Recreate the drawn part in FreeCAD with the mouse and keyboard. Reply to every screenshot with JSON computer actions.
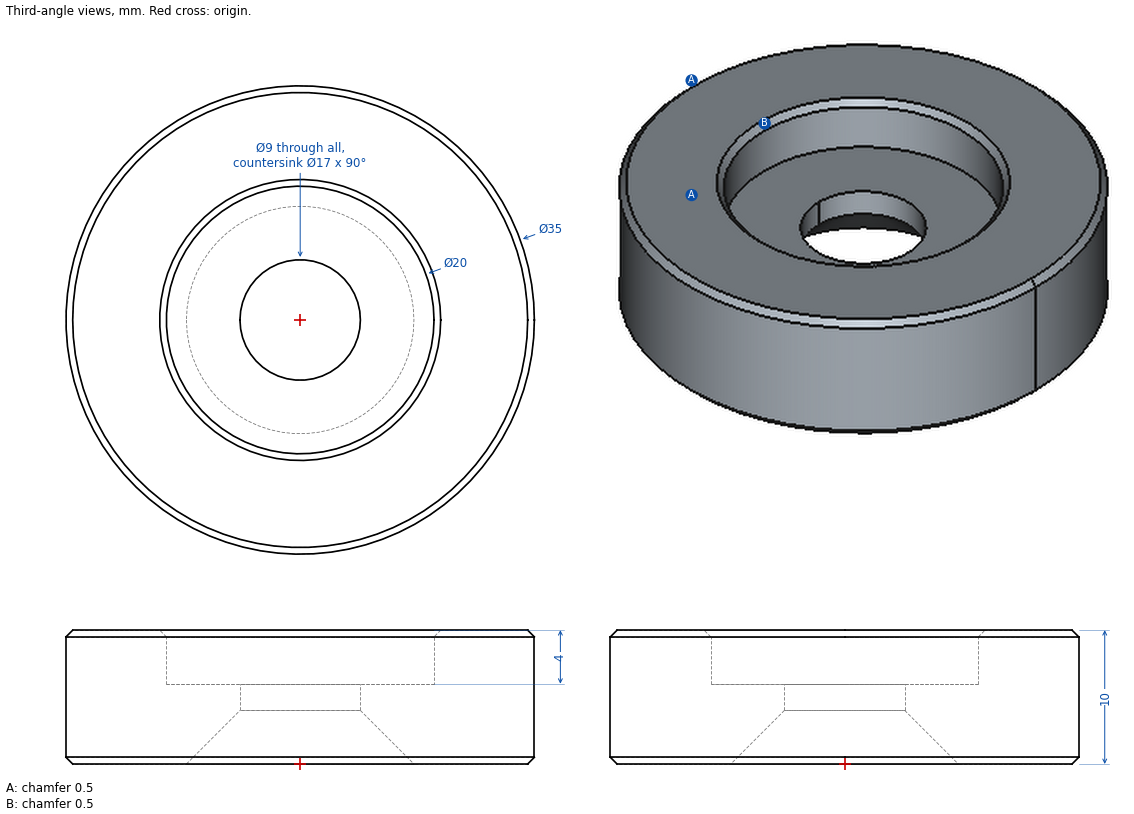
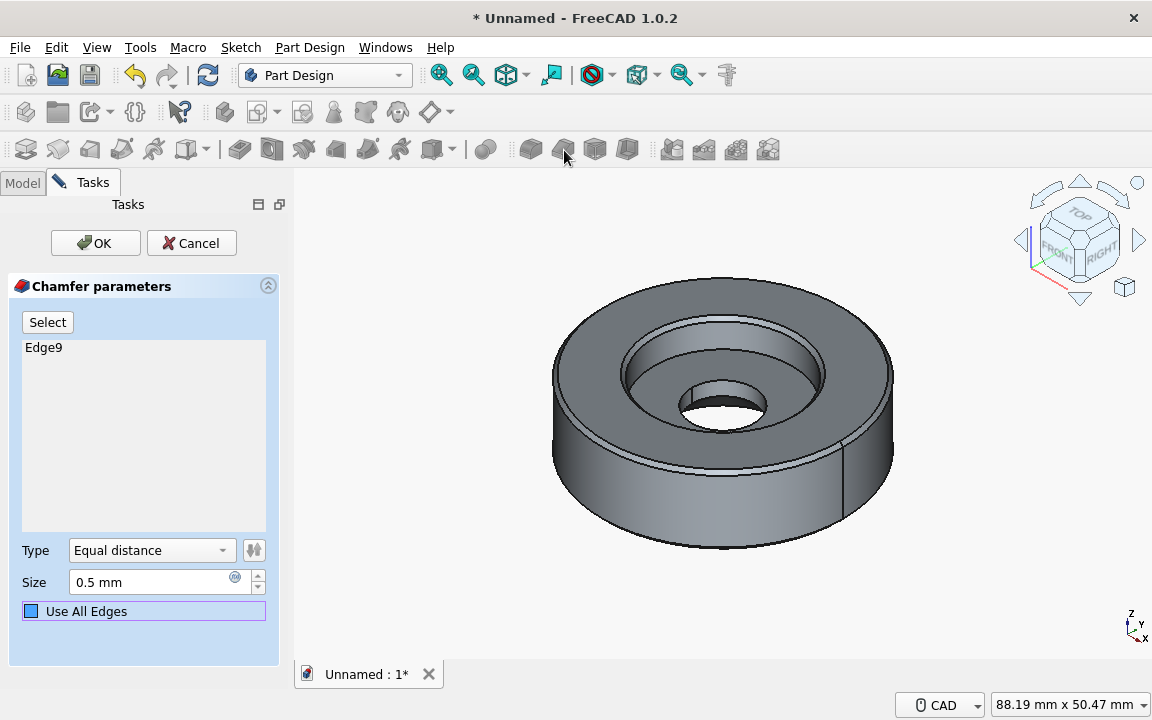
{"action": "left_click", "coordinate": [96, 243]}